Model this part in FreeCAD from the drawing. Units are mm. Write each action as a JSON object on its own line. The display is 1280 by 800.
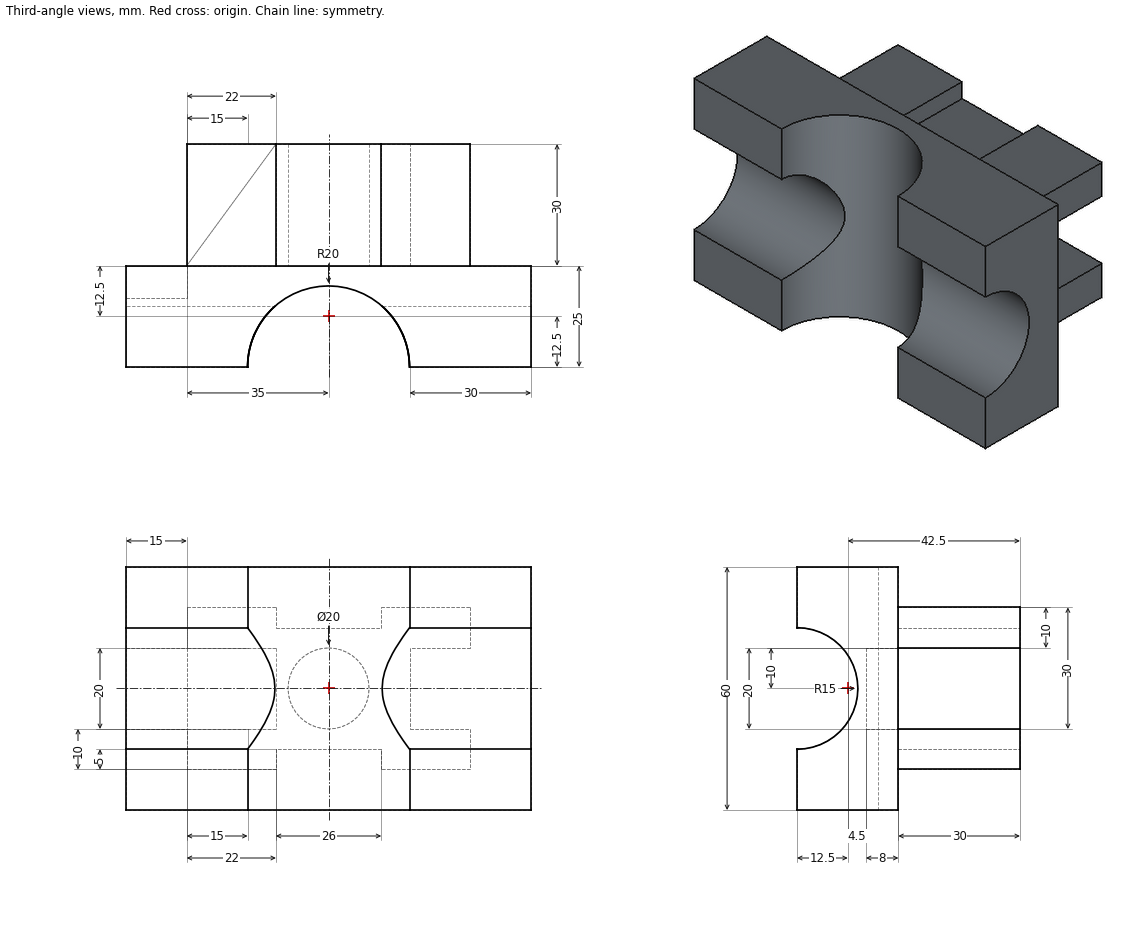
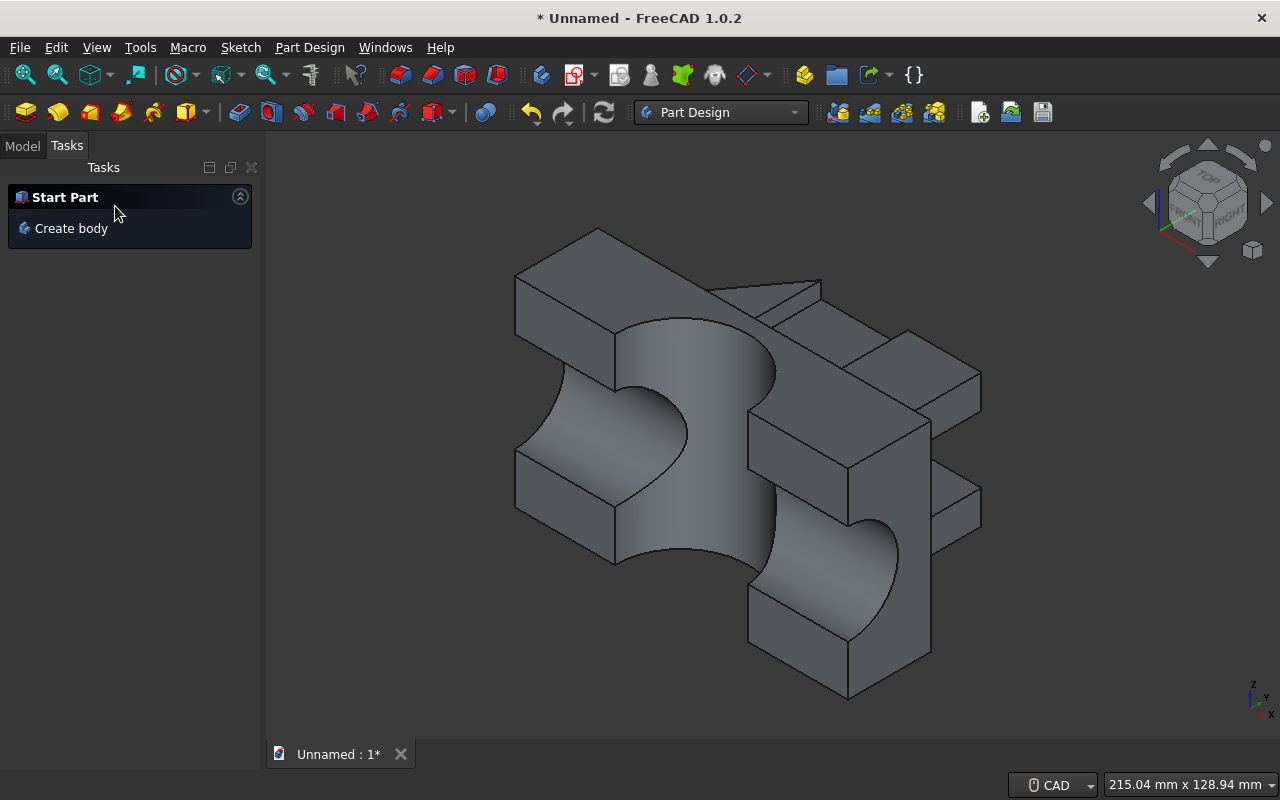
{"action": "left_click", "coordinate": [895, 379]}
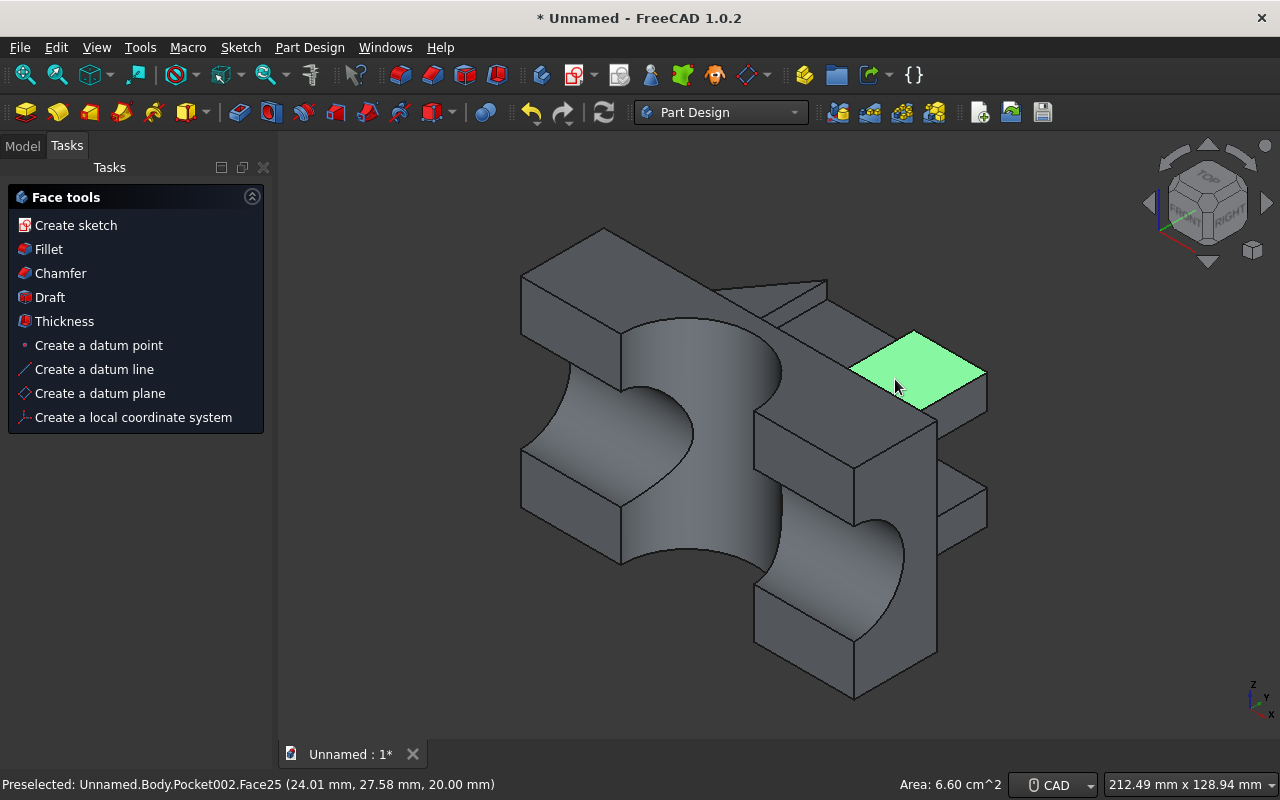
{"action": "left_click", "coordinate": [574, 76]}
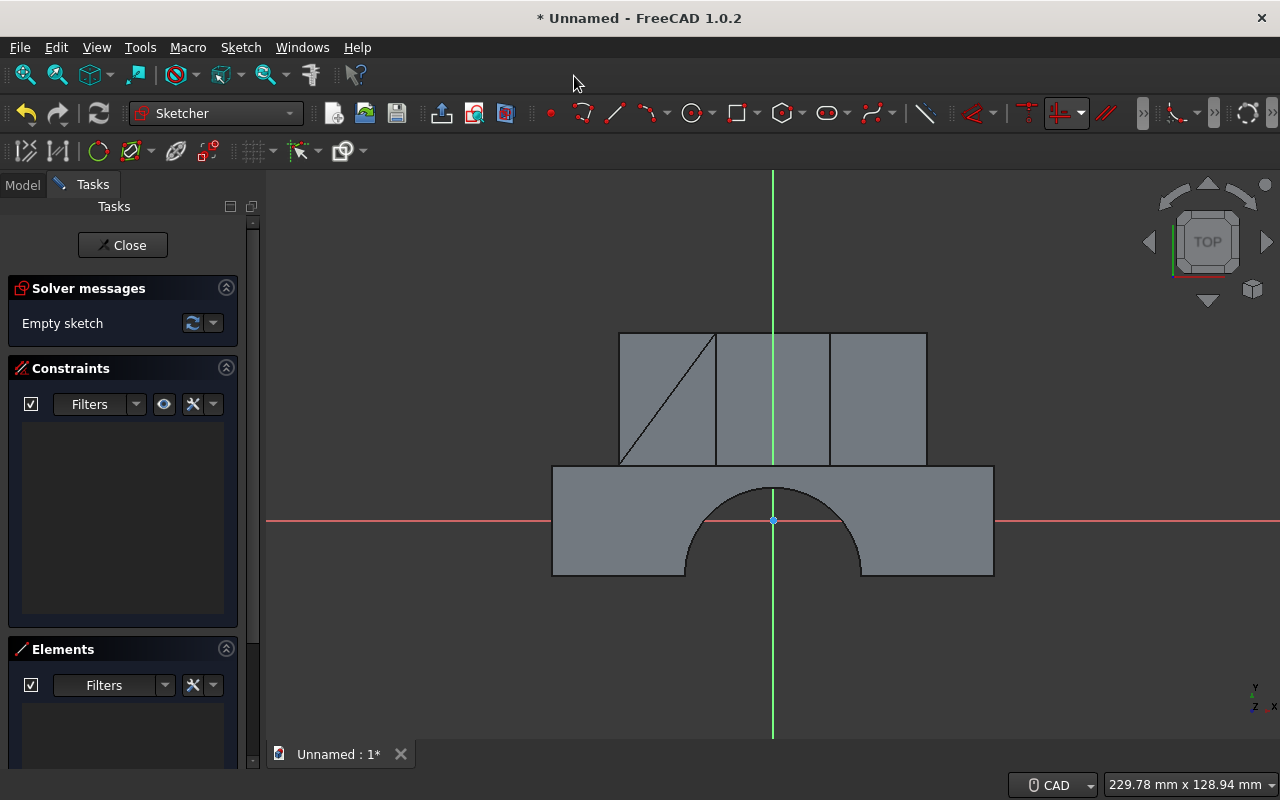
{"action": "left_click", "coordinate": [506, 114]}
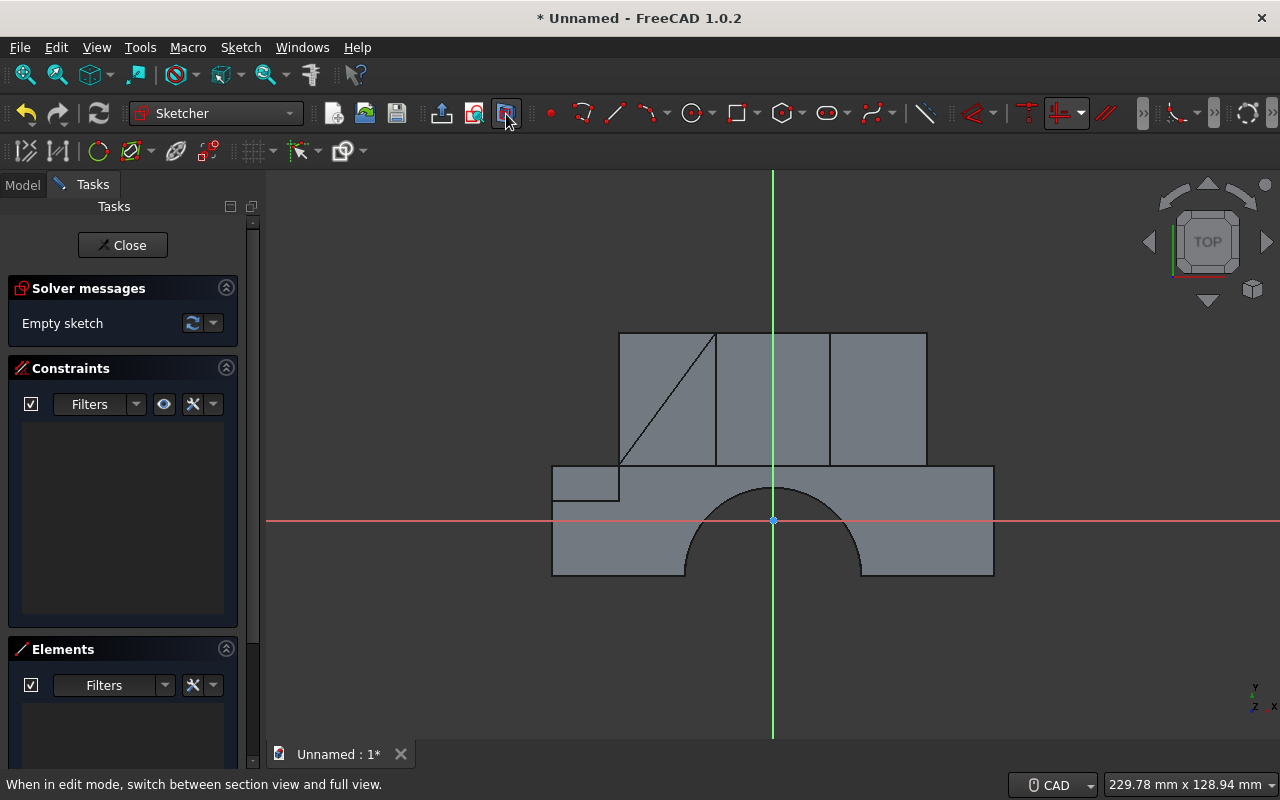
{"action": "scroll", "coordinate": [685, 393], "scroll_direction": "up", "scroll_amount": 3}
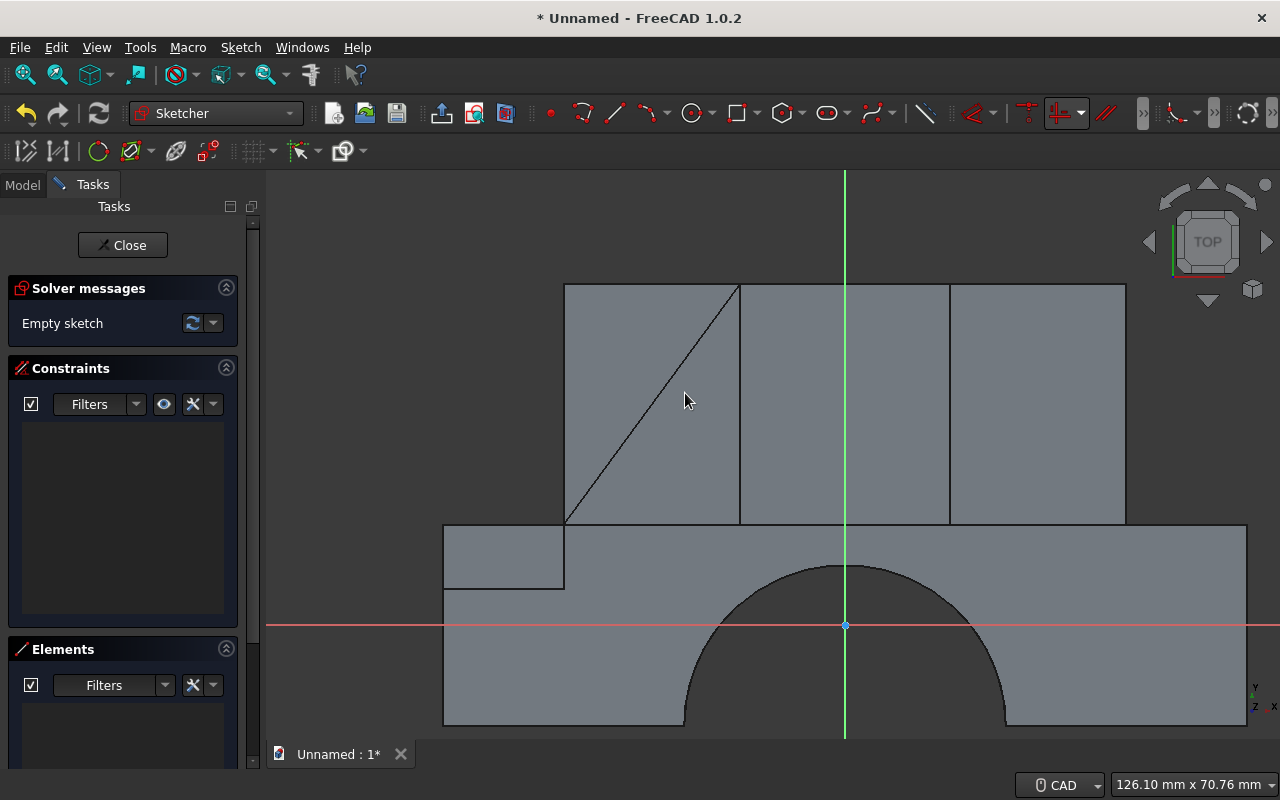
{"action": "left_click", "coordinate": [584, 114]}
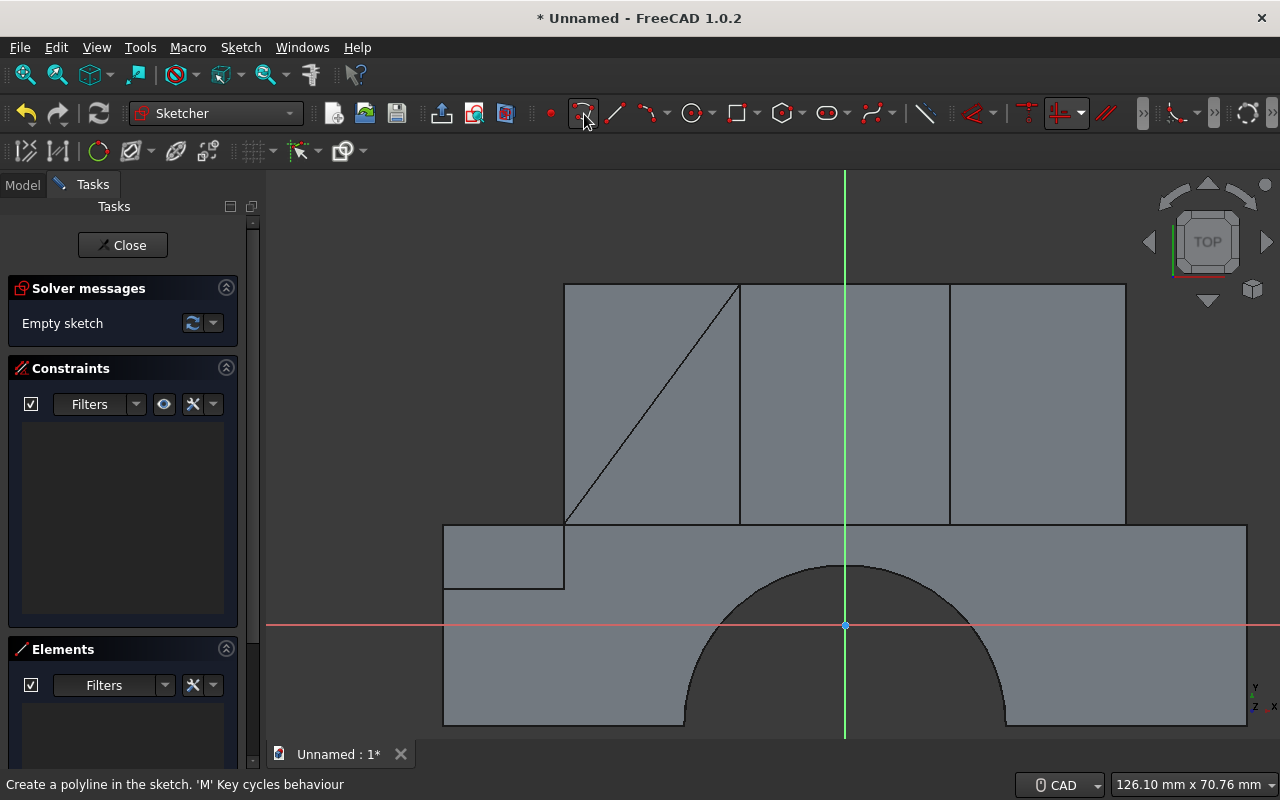
{"action": "left_click", "coordinate": [564, 525]}
{"action": "left_click", "coordinate": [740, 284]}
{"action": "left_click", "coordinate": [564, 284]}
{"action": "left_click", "coordinate": [564, 526]}
{"action": "key", "text": "Escape"}
{"action": "key", "text": "Escape"}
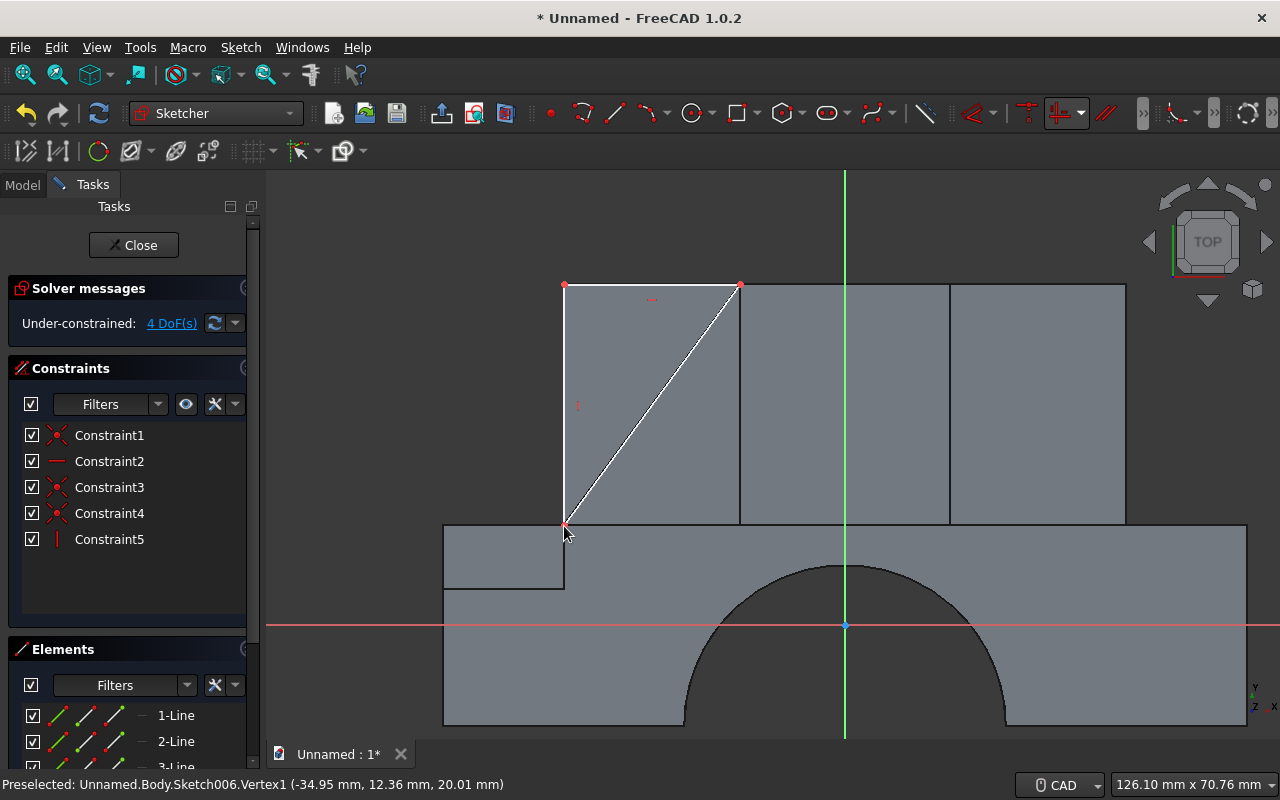
{"action": "key", "text": "d"}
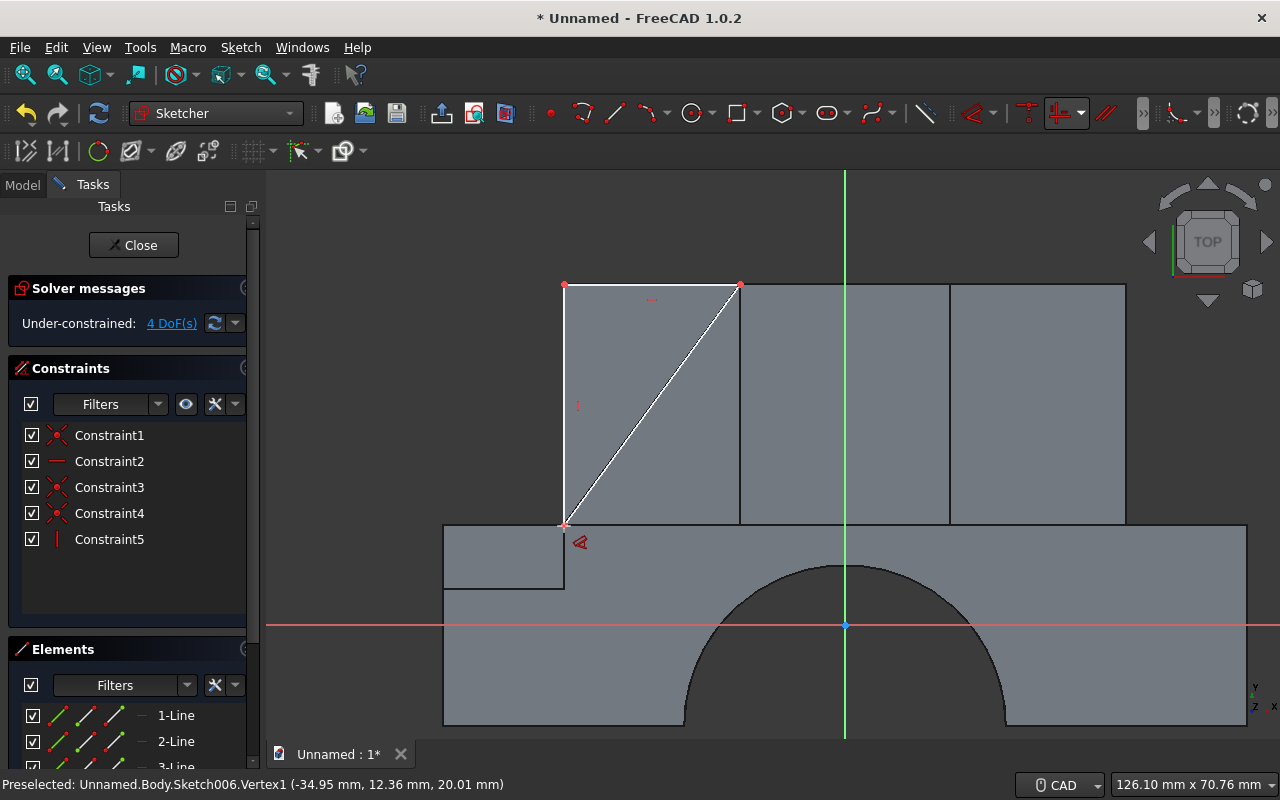
{"action": "left_click", "coordinate": [687, 285]}
{"action": "left_click", "coordinate": [652, 251]}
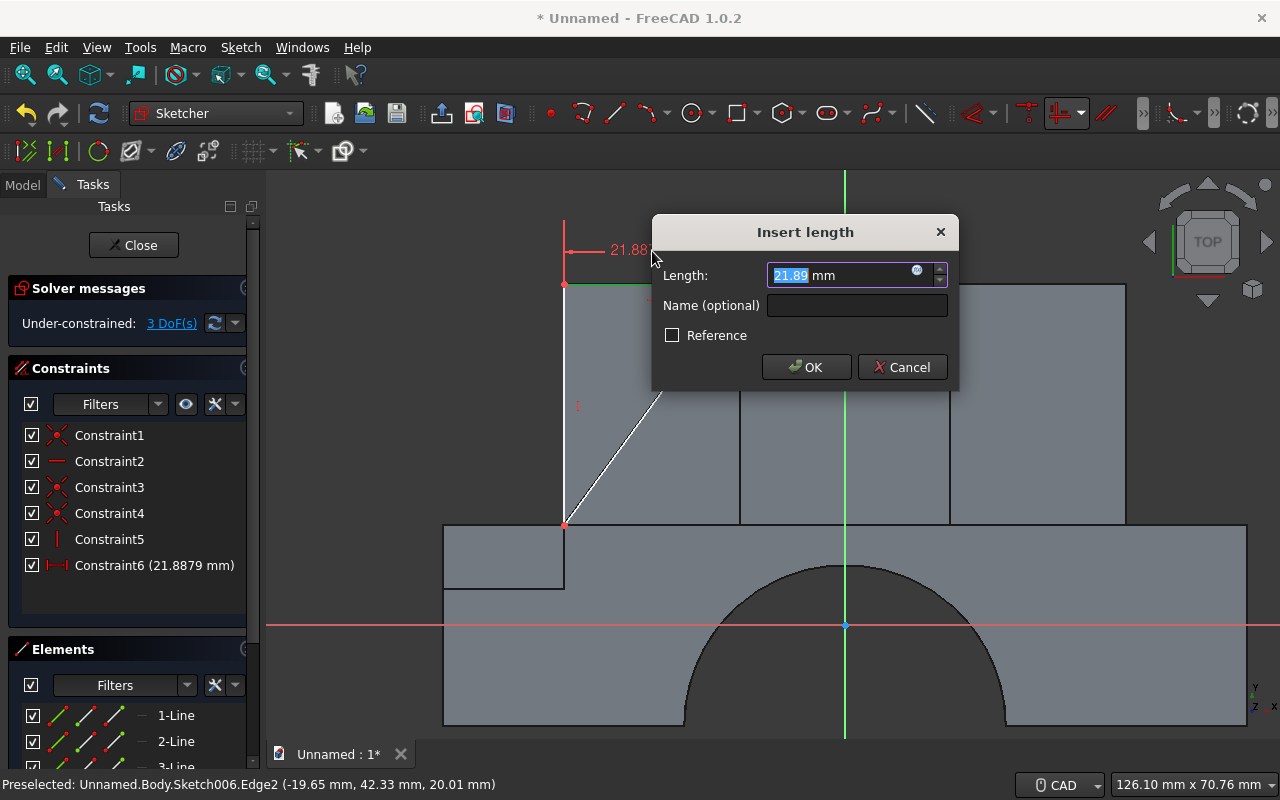
{"action": "type", "text": "22"}
{"action": "key", "text": "Return"}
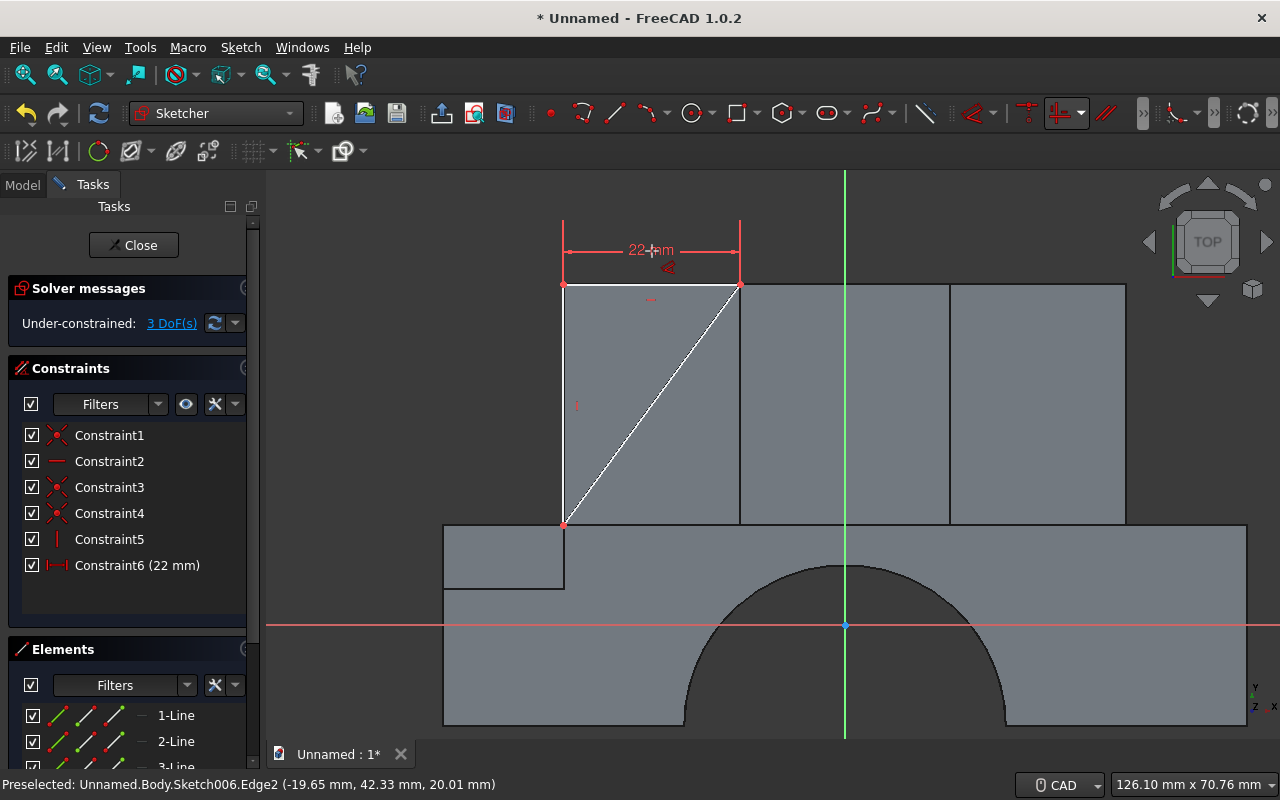
{"action": "left_click", "coordinate": [563, 357]}
{"action": "left_click", "coordinate": [529, 406]}